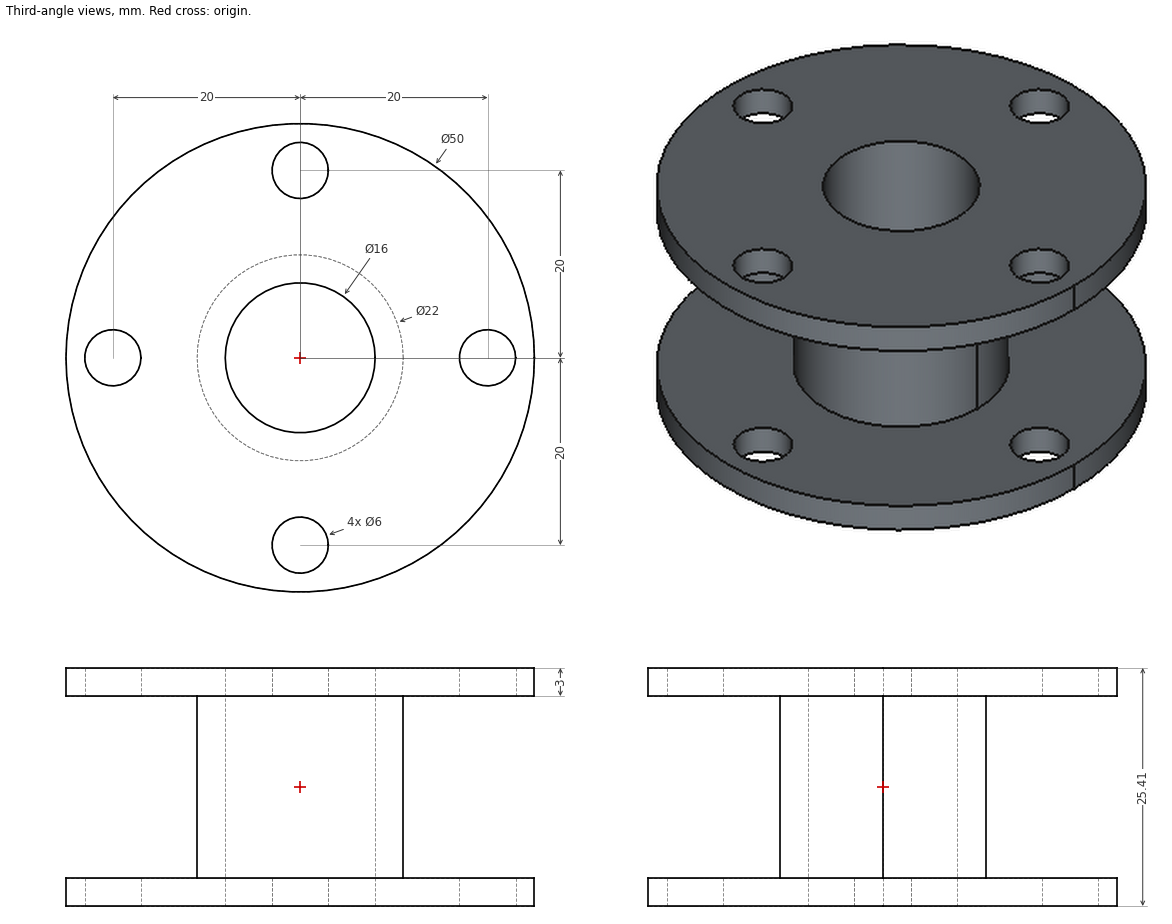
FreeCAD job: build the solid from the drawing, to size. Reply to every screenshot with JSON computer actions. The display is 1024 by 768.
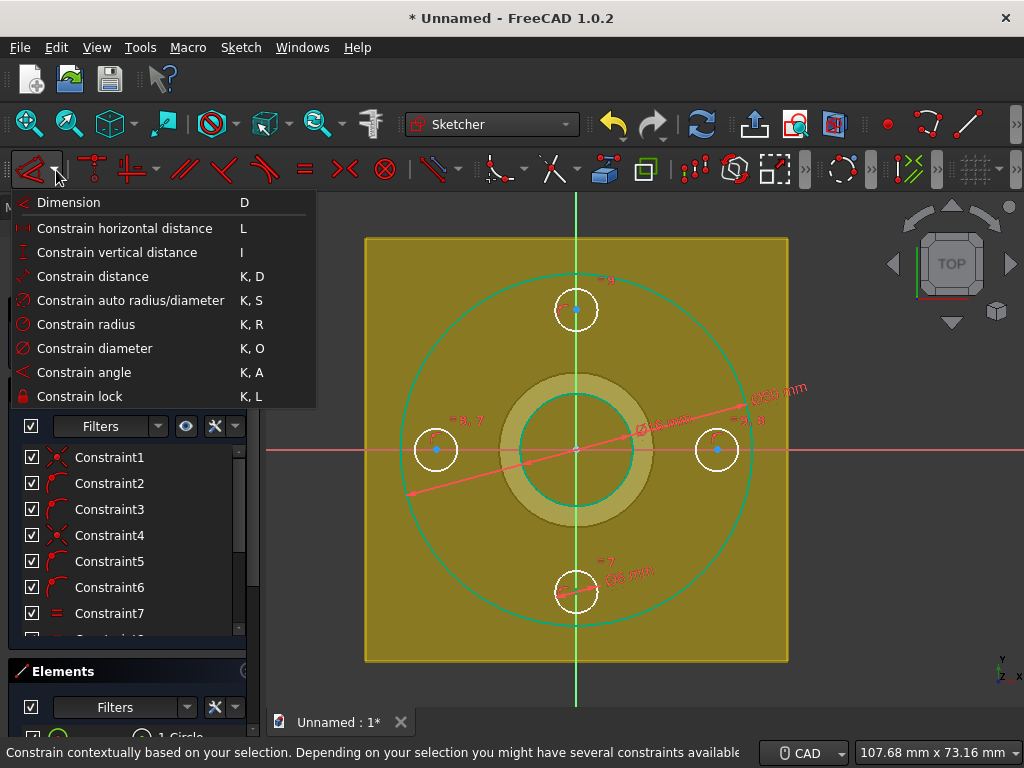
{"action": "left_click", "coordinate": [164, 252]}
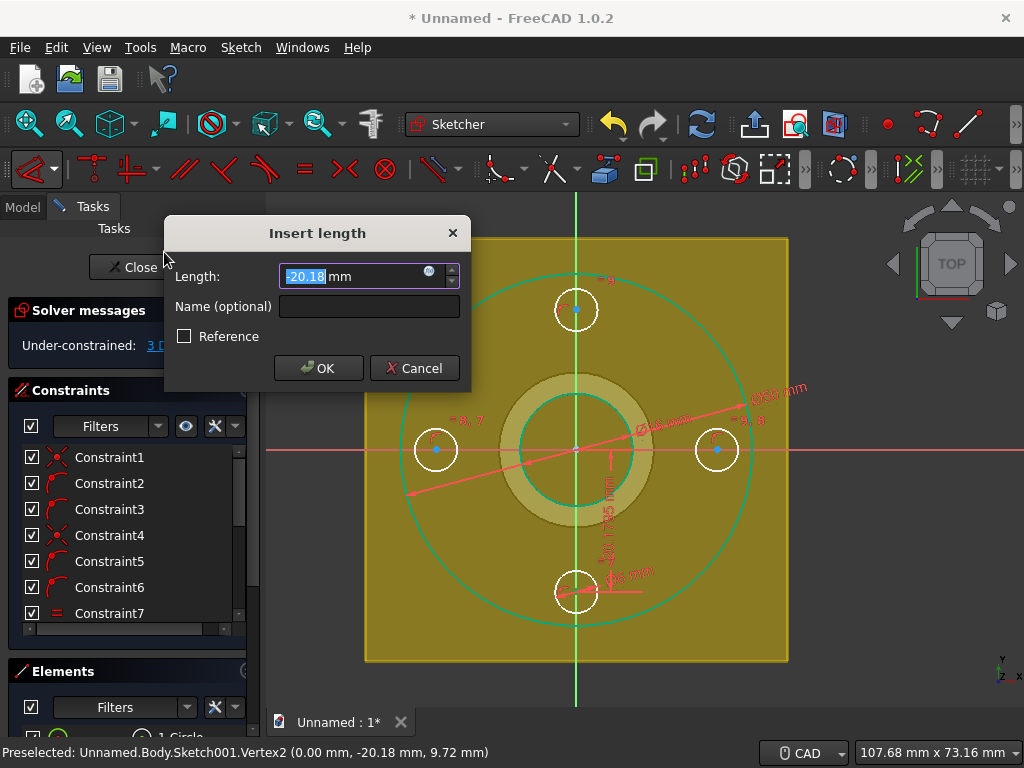
{"action": "type", "text": "-20"}
{"action": "key", "text": "Return"}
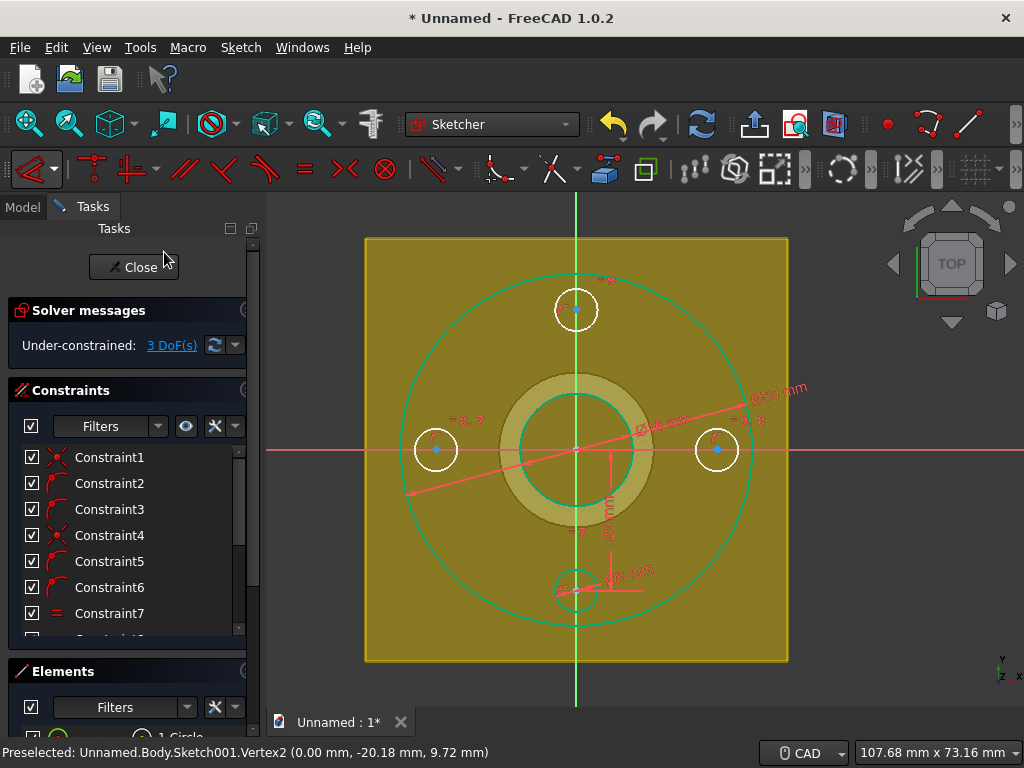
{"action": "left_click", "coordinate": [436, 450]}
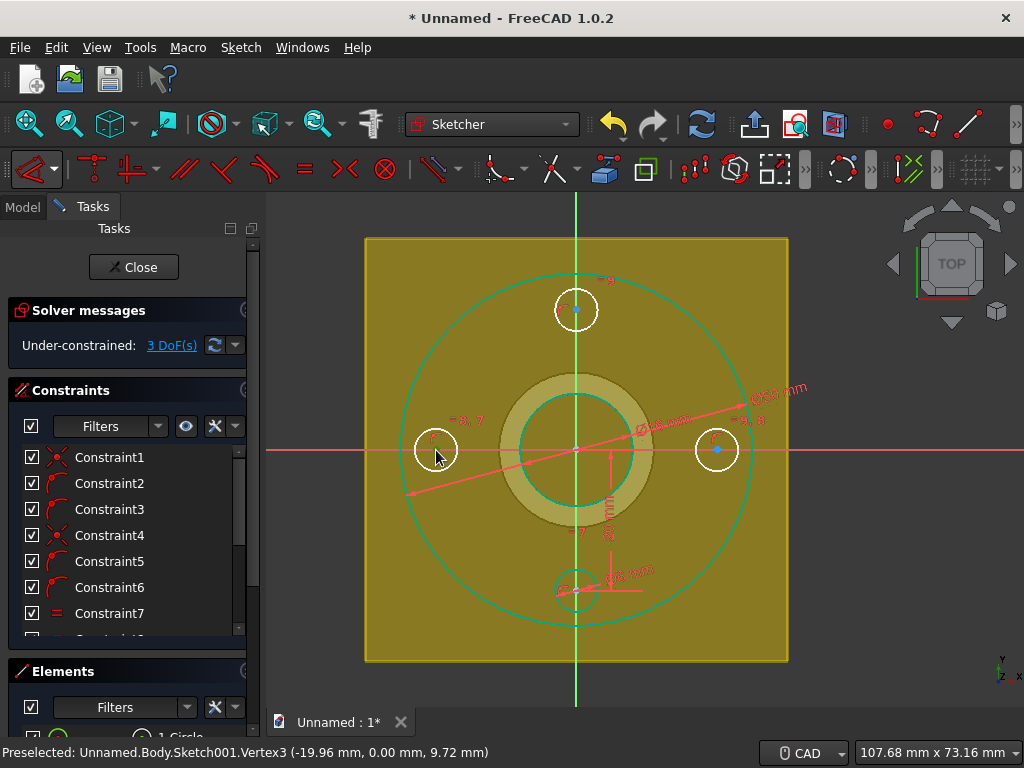
{"action": "left_click", "coordinate": [56, 170]}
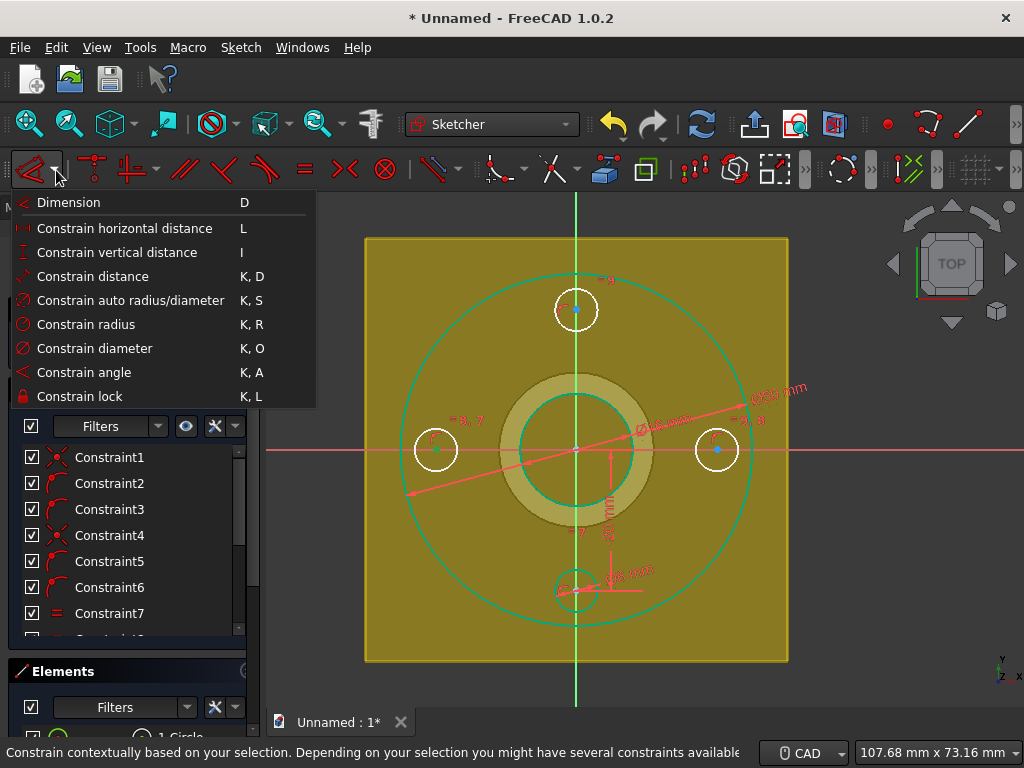
{"action": "left_click", "coordinate": [164, 228]}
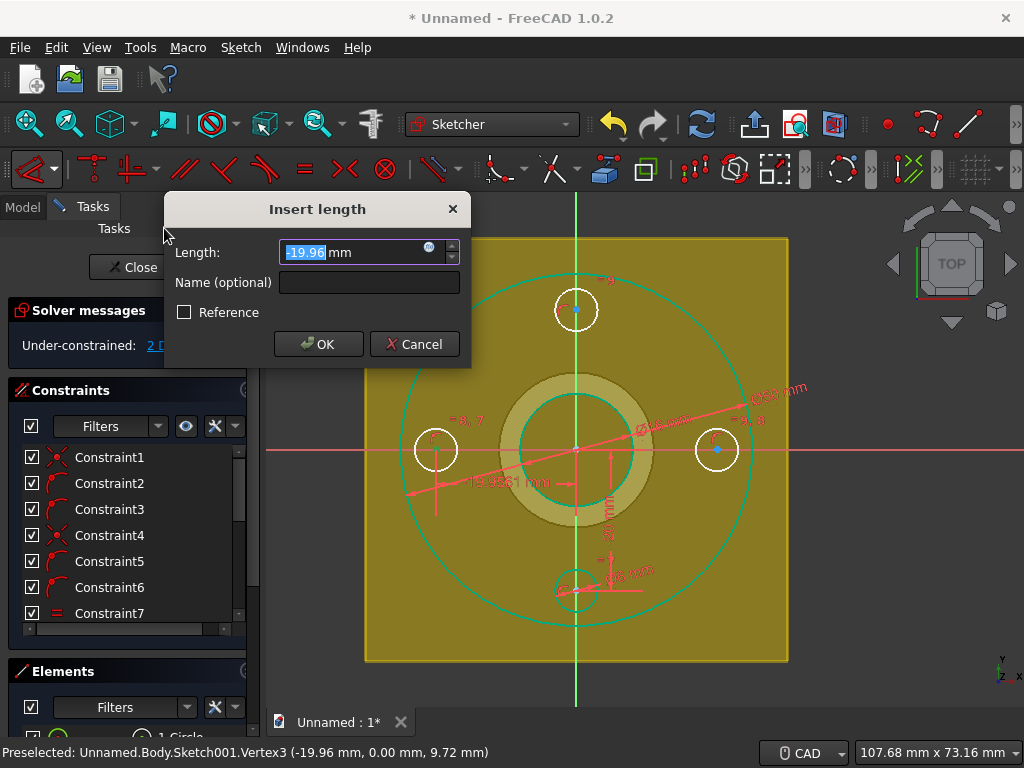
{"action": "type", "text": "-20"}
{"action": "key", "text": "Return"}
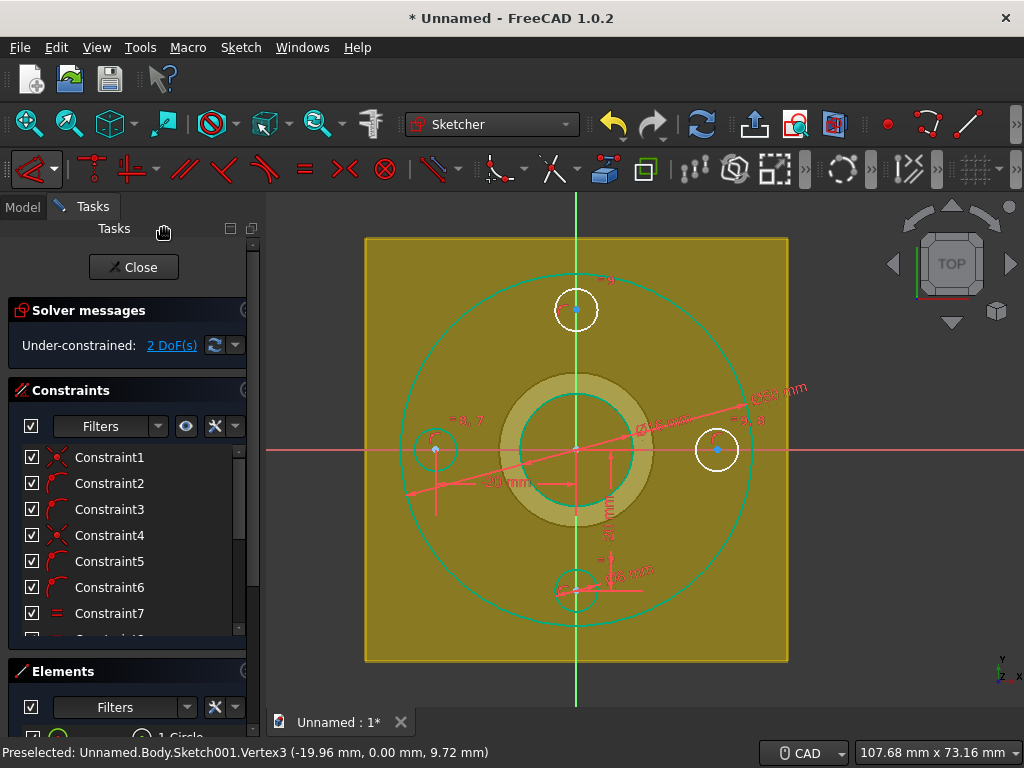
{"action": "left_click", "coordinate": [717, 450]}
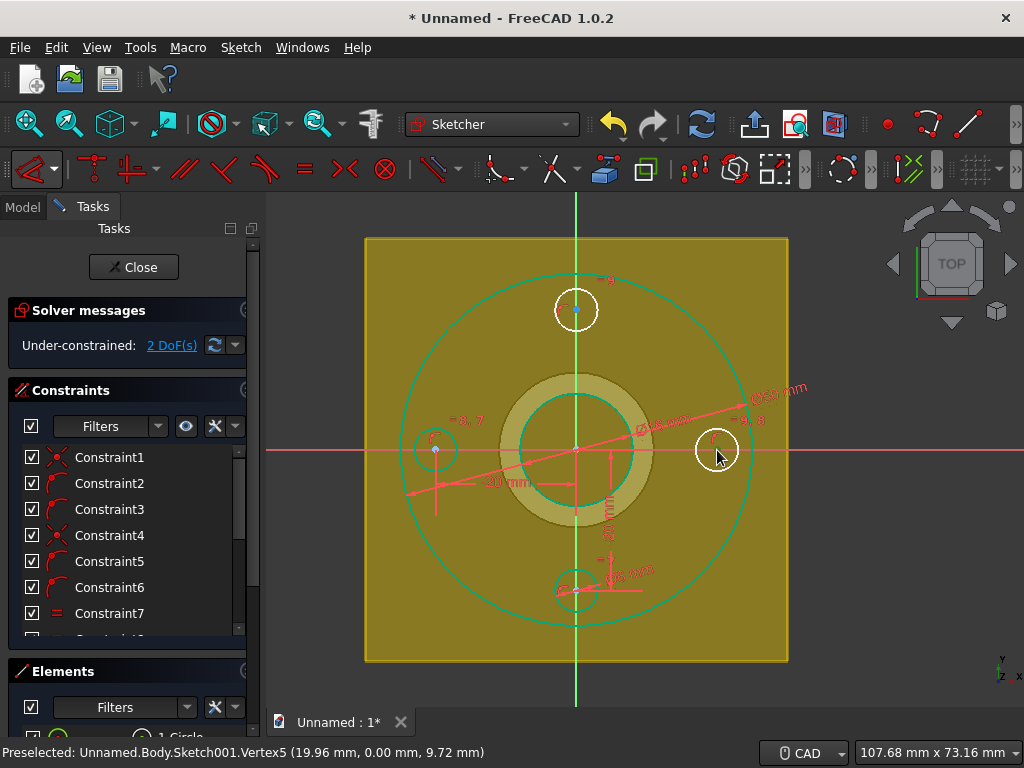
{"action": "left_click", "coordinate": [56, 170]}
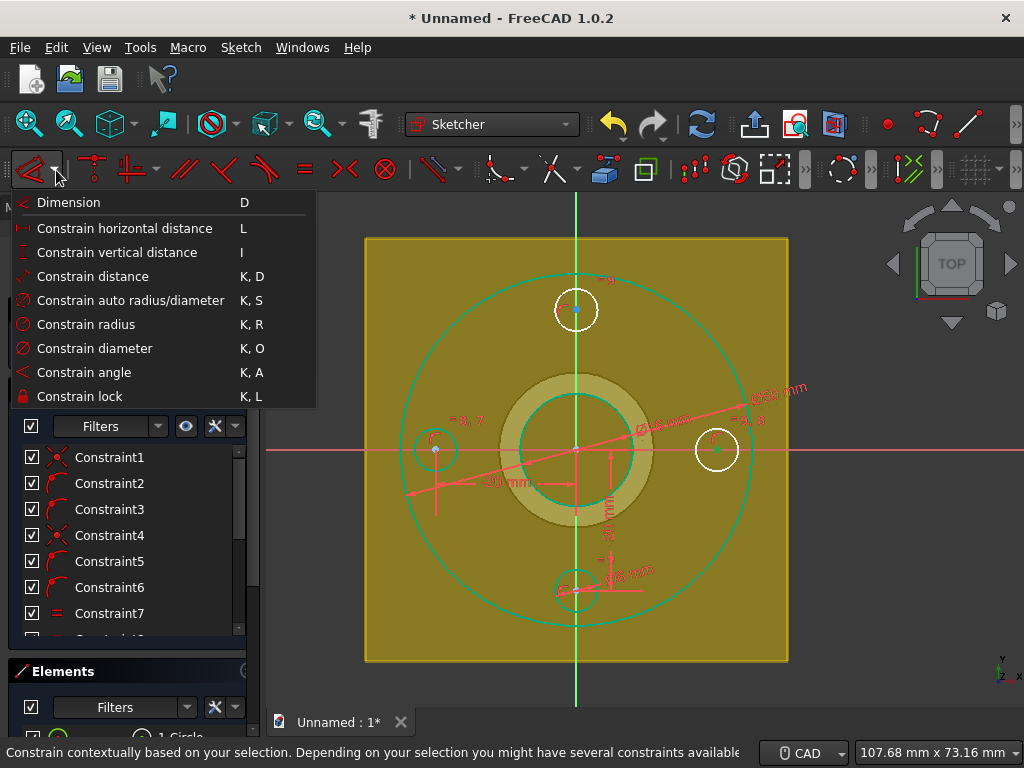
{"action": "left_click", "coordinate": [164, 228]}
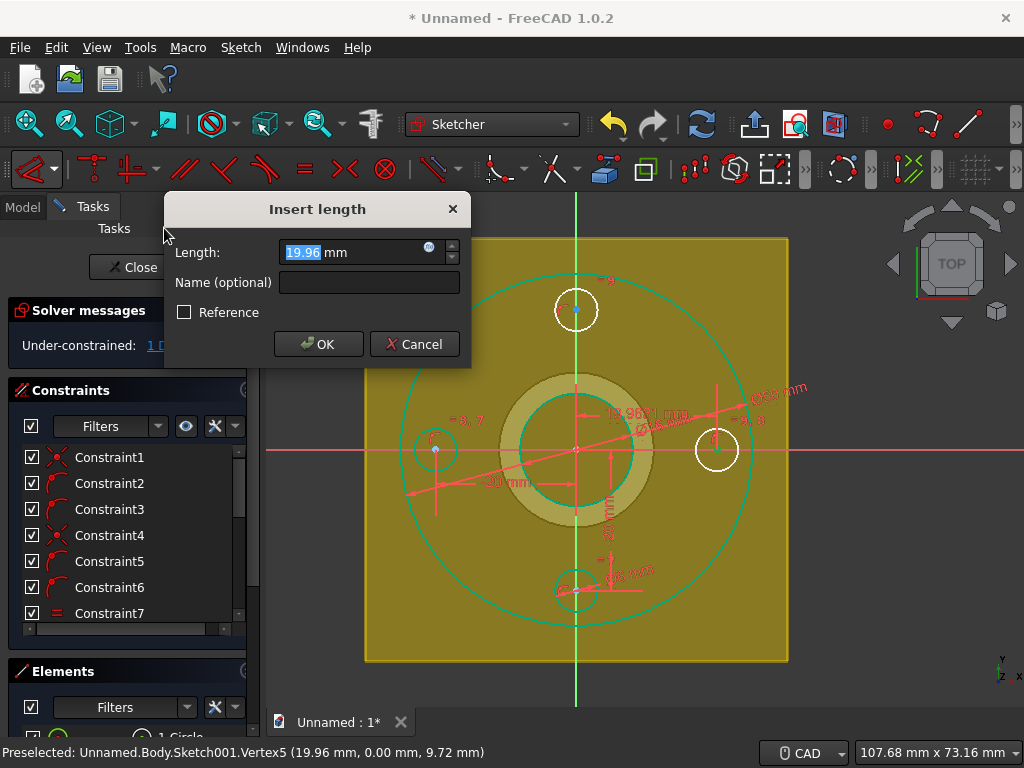
{"action": "type", "text": "20"}
{"action": "key", "text": "Return"}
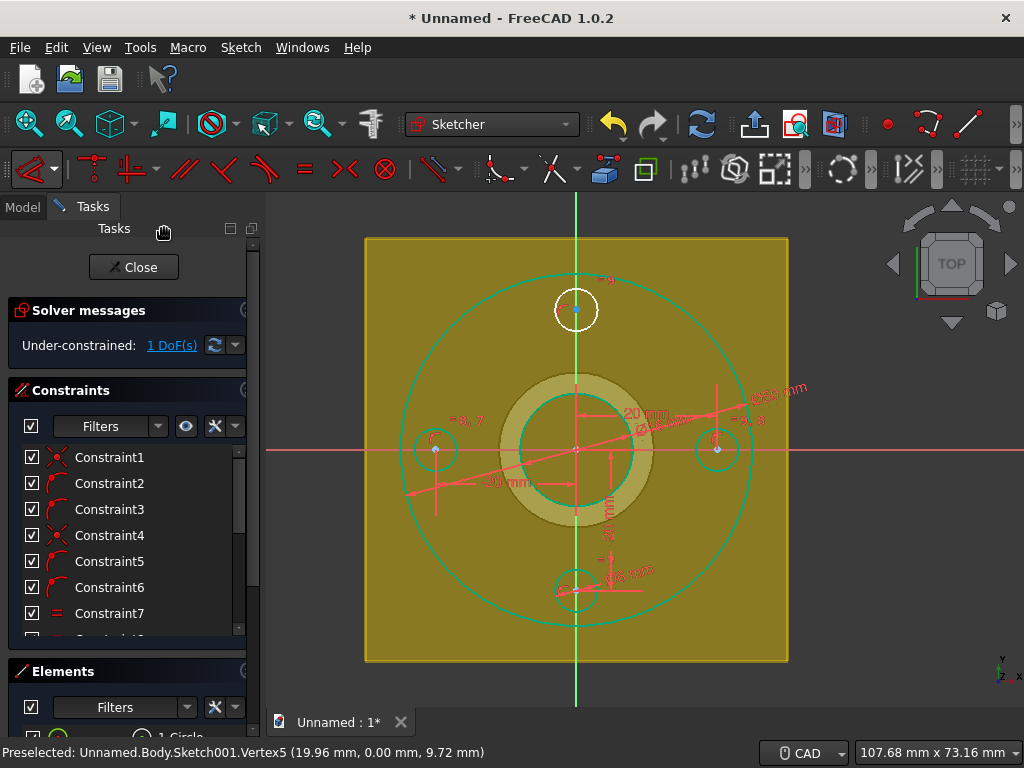
{"action": "left_click", "coordinate": [576, 310]}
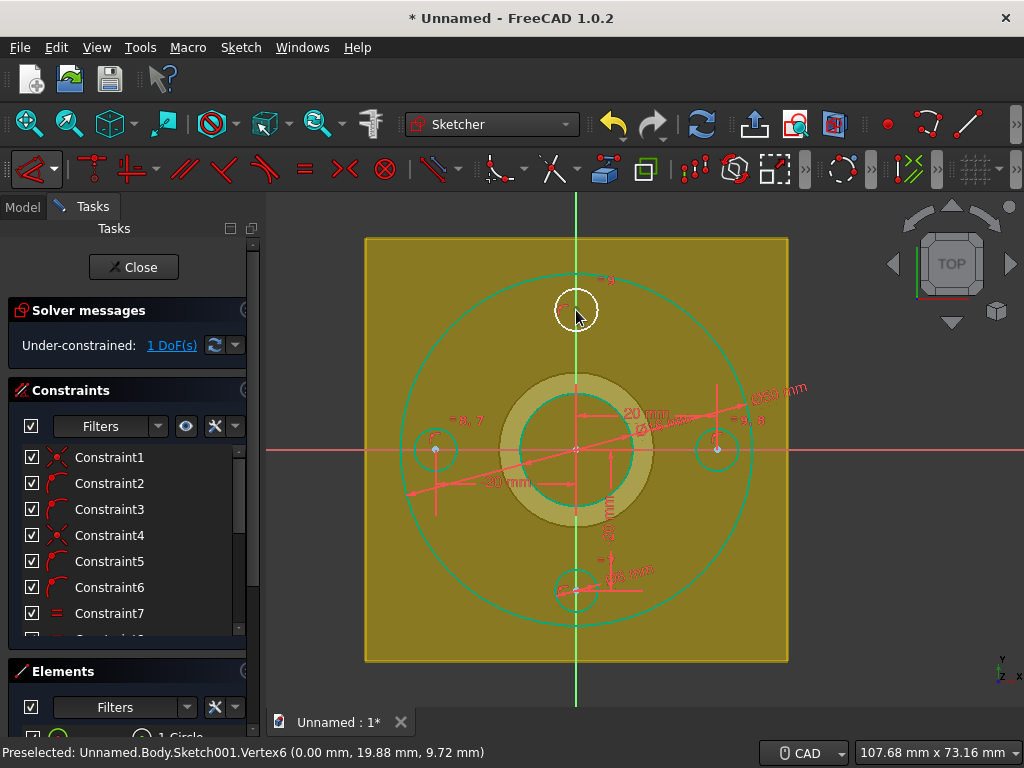
{"action": "left_click", "coordinate": [56, 170]}